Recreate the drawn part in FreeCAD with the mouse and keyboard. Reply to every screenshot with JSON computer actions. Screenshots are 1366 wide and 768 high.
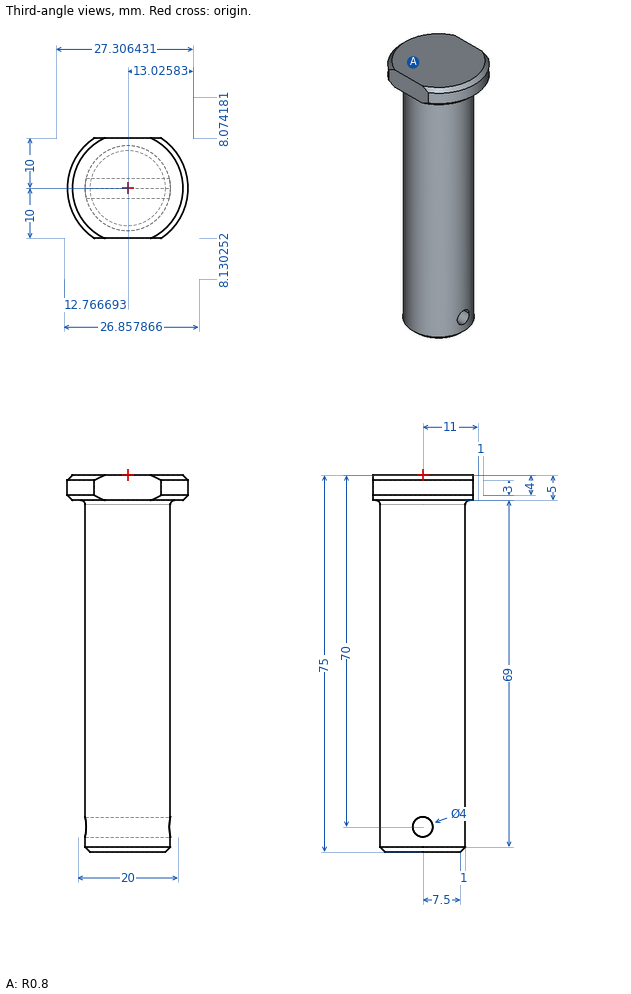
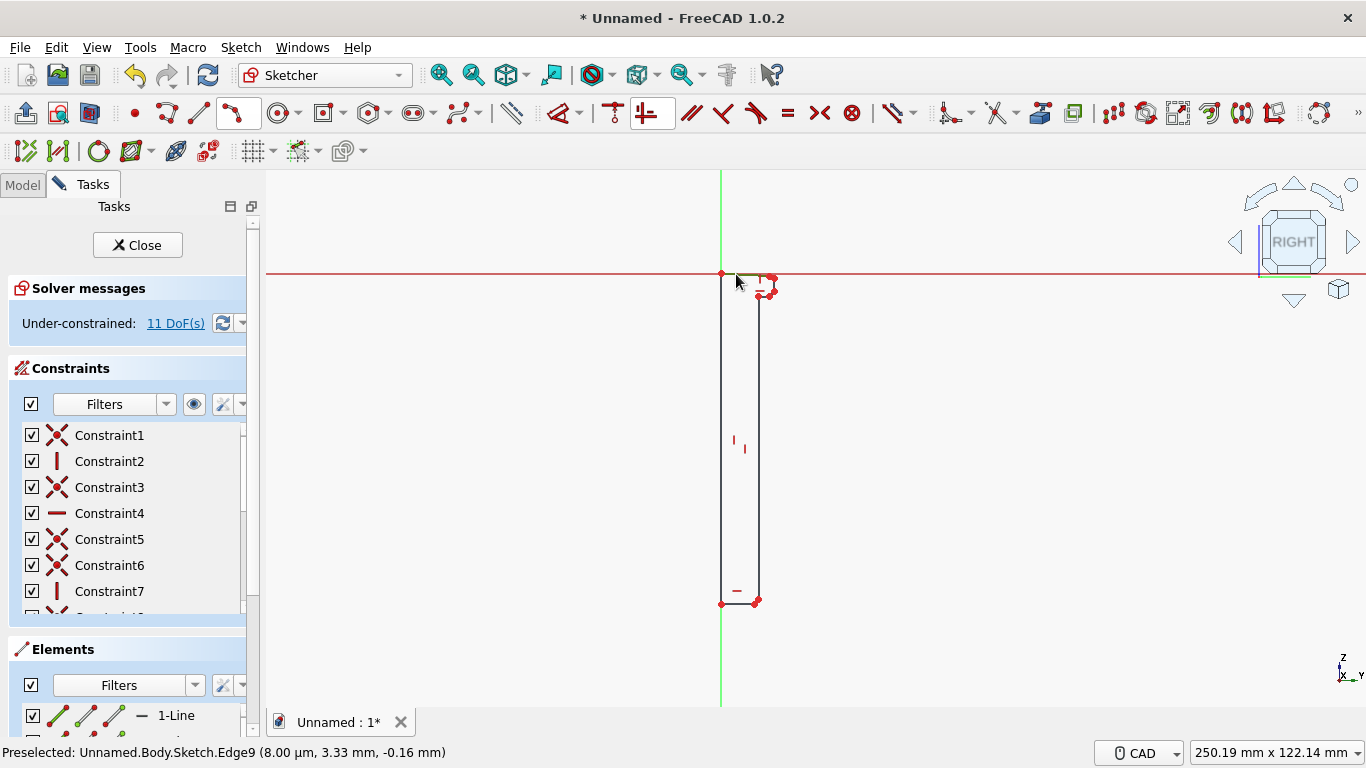
{"action": "key", "text": "h"}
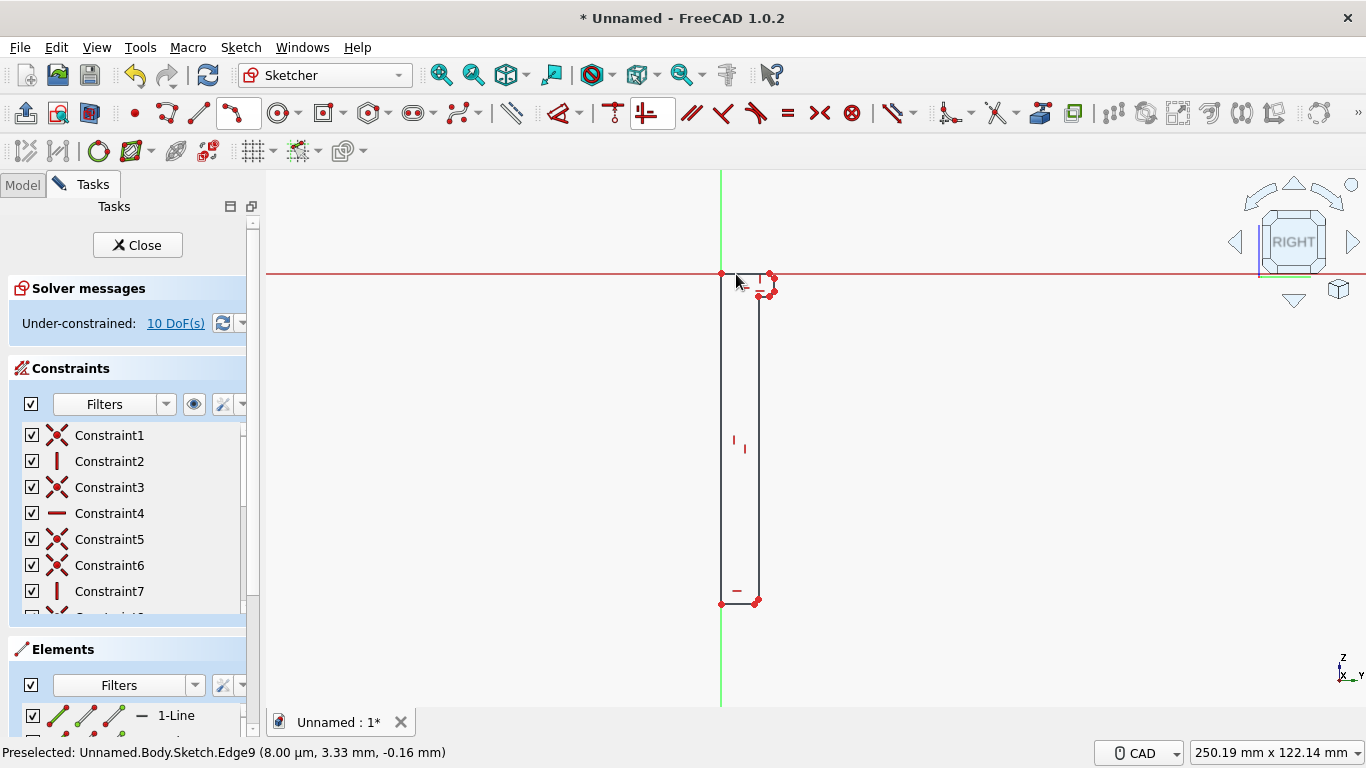
{"action": "left_click", "coordinate": [558, 114]}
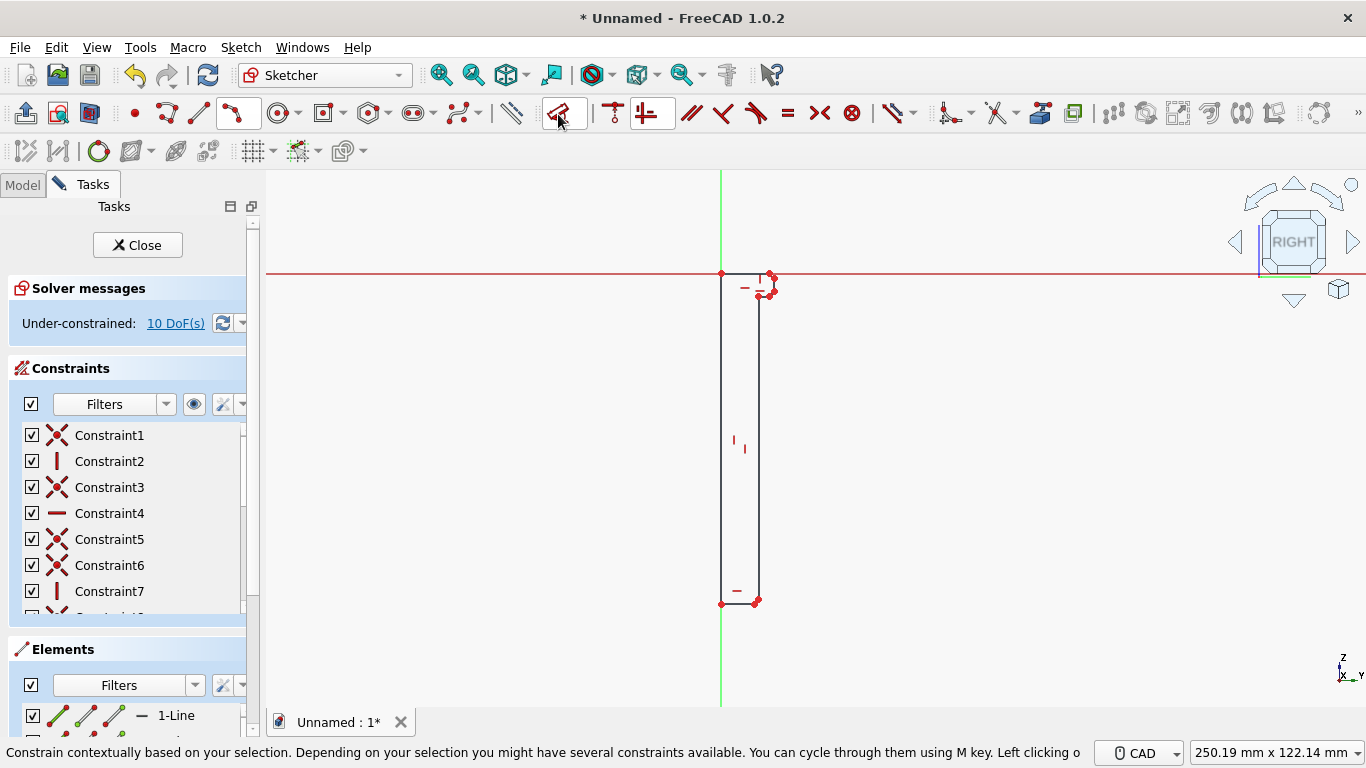
{"action": "scroll", "coordinate": [774, 285], "scroll_direction": "up", "scroll_amount": 6}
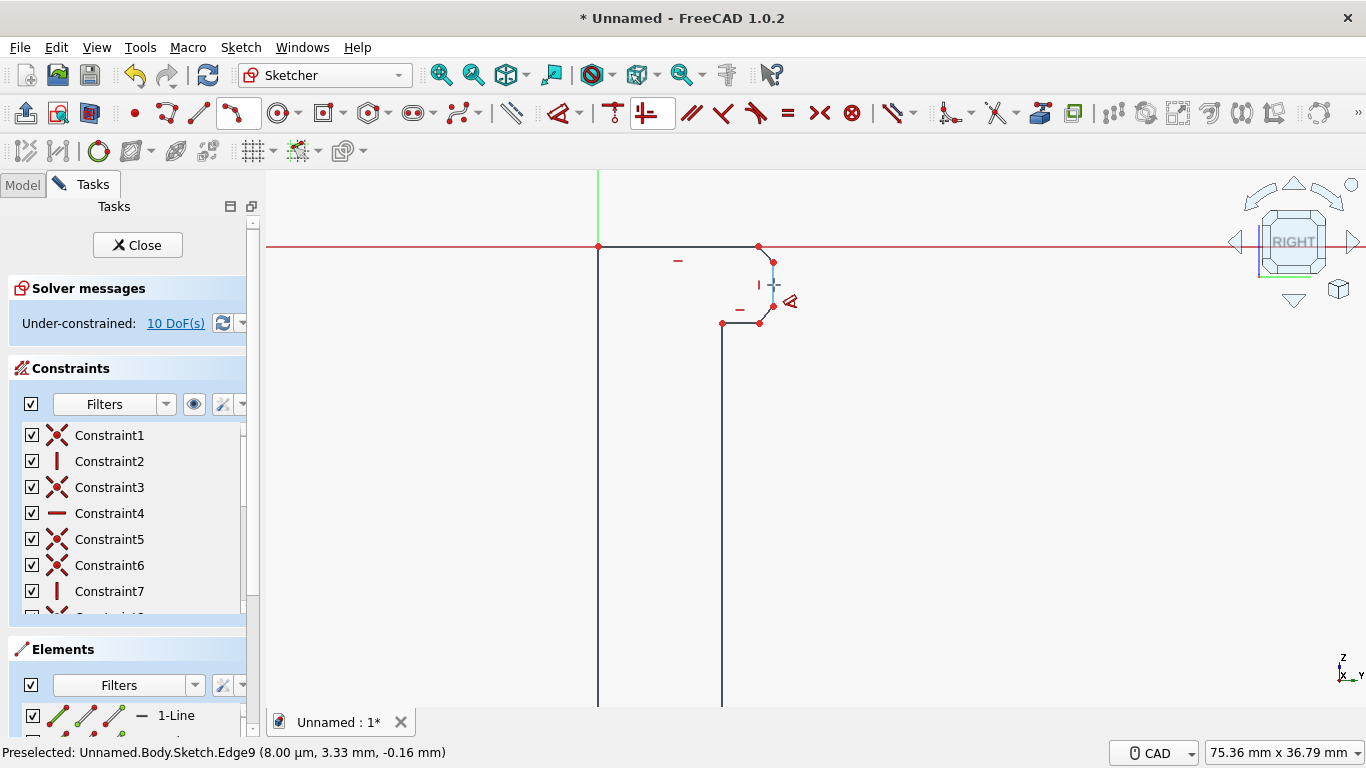
{"action": "left_click", "coordinate": [773, 284]}
{"action": "left_click", "coordinate": [807, 284]}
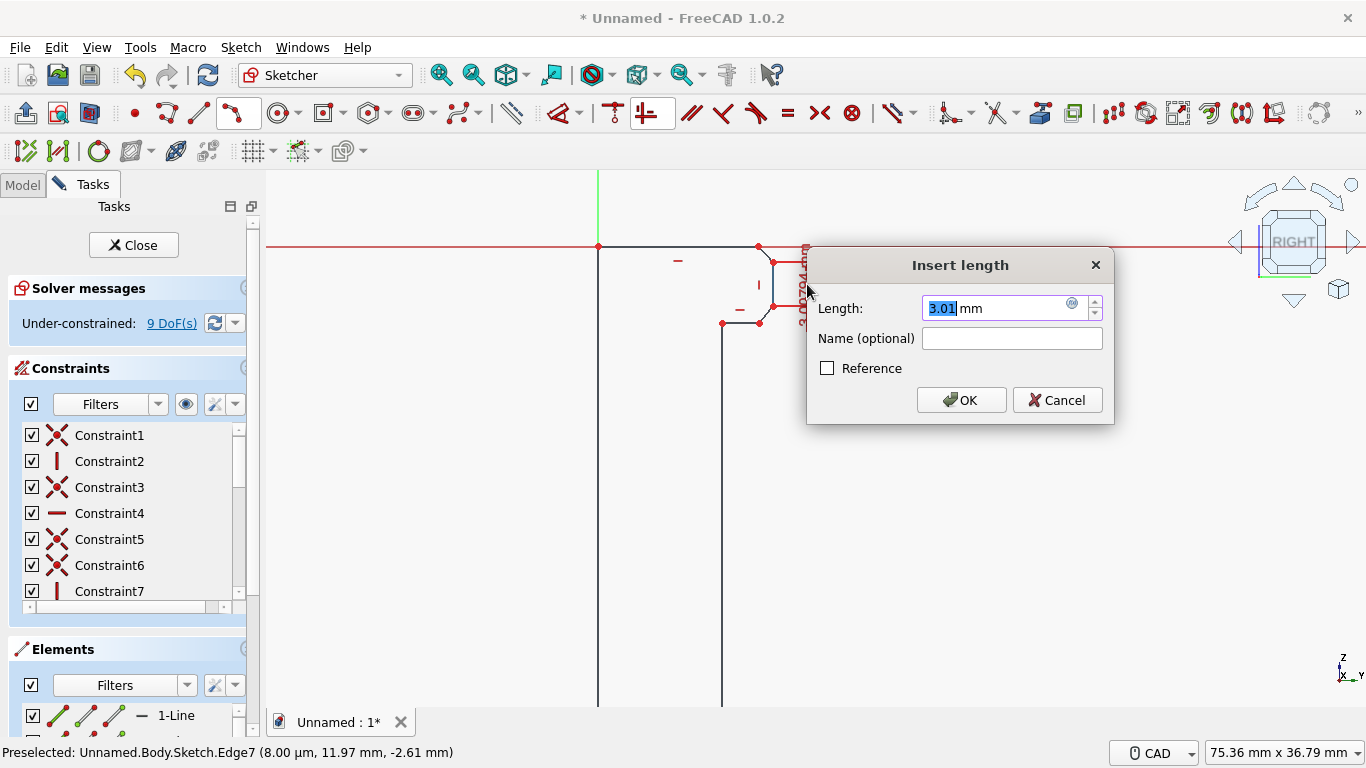
{"action": "type", "text": "3"}
{"action": "key", "text": "Return"}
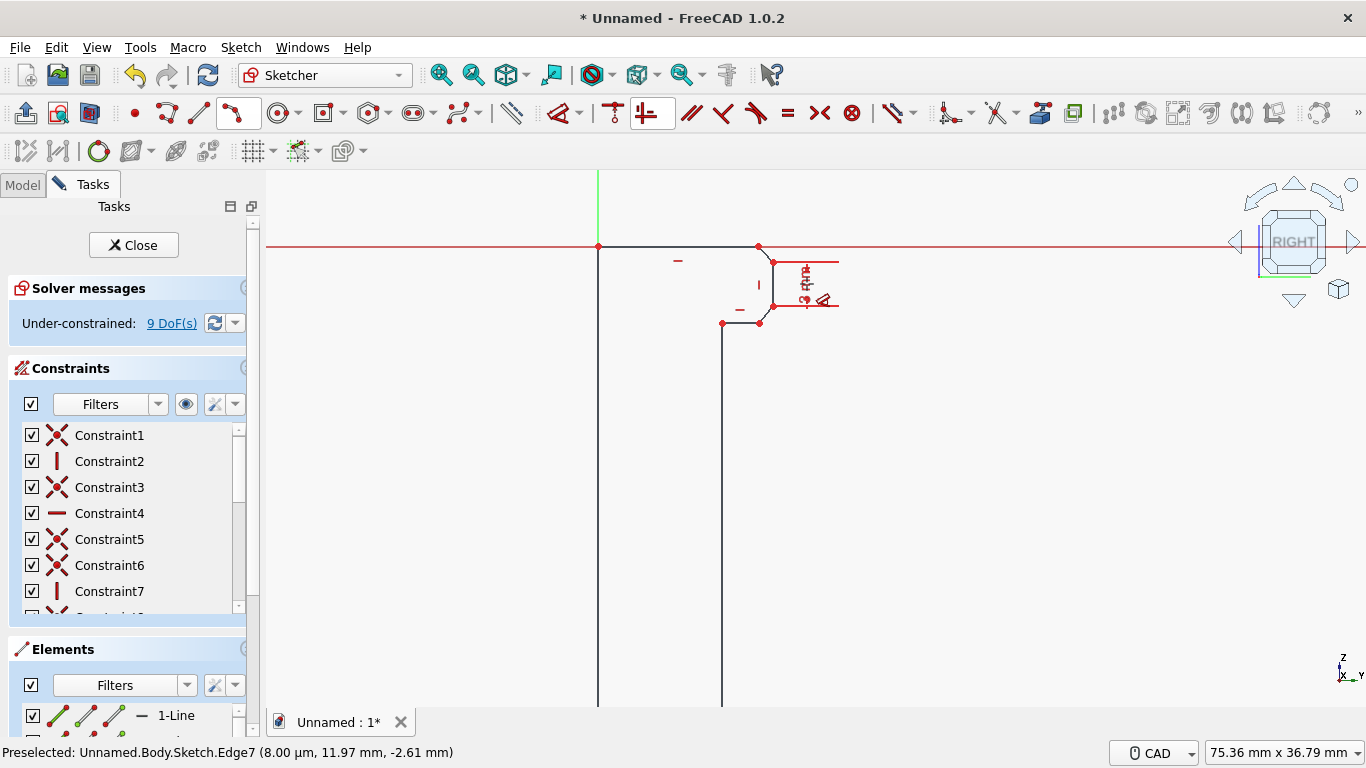
{"action": "scroll", "coordinate": [774, 285], "scroll_direction": "down", "scroll_amount": 6}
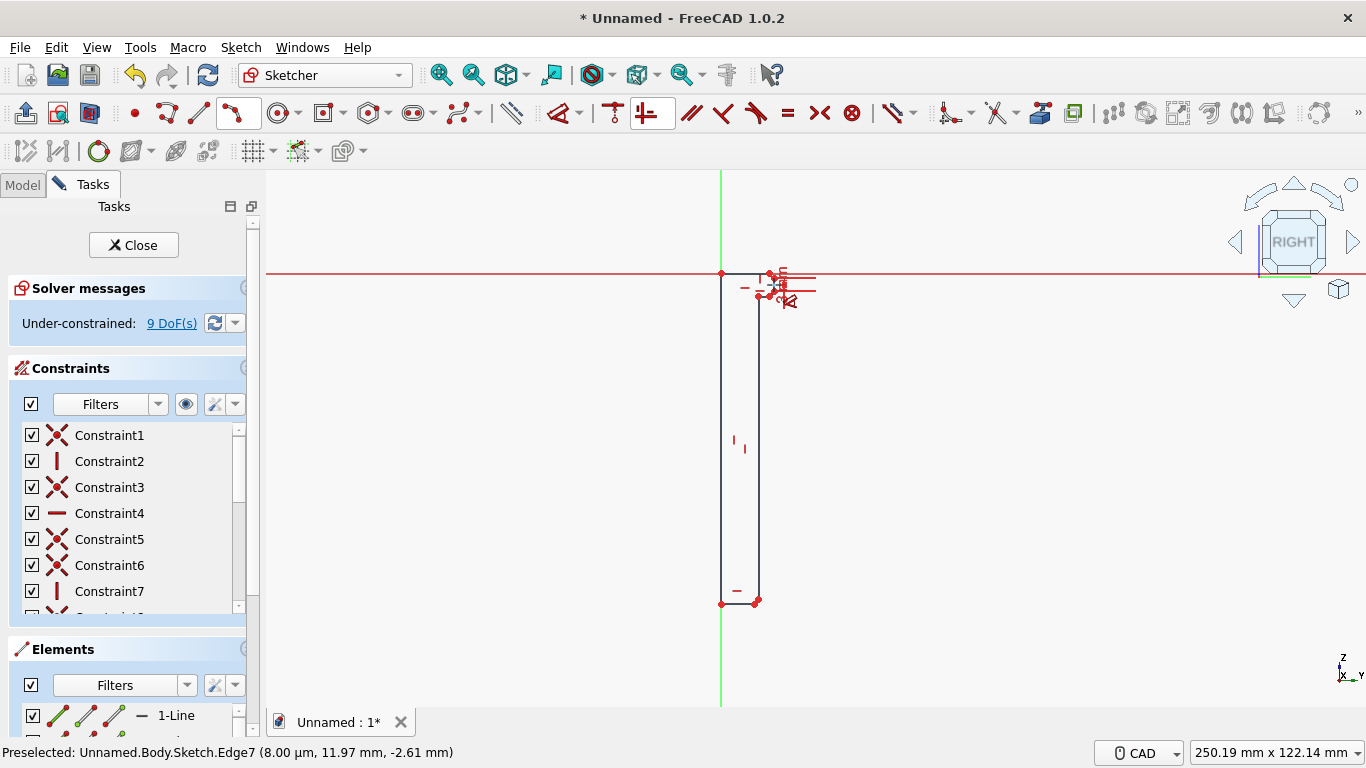
{"action": "left_click", "coordinate": [721, 373]}
{"action": "left_click", "coordinate": [687, 439]}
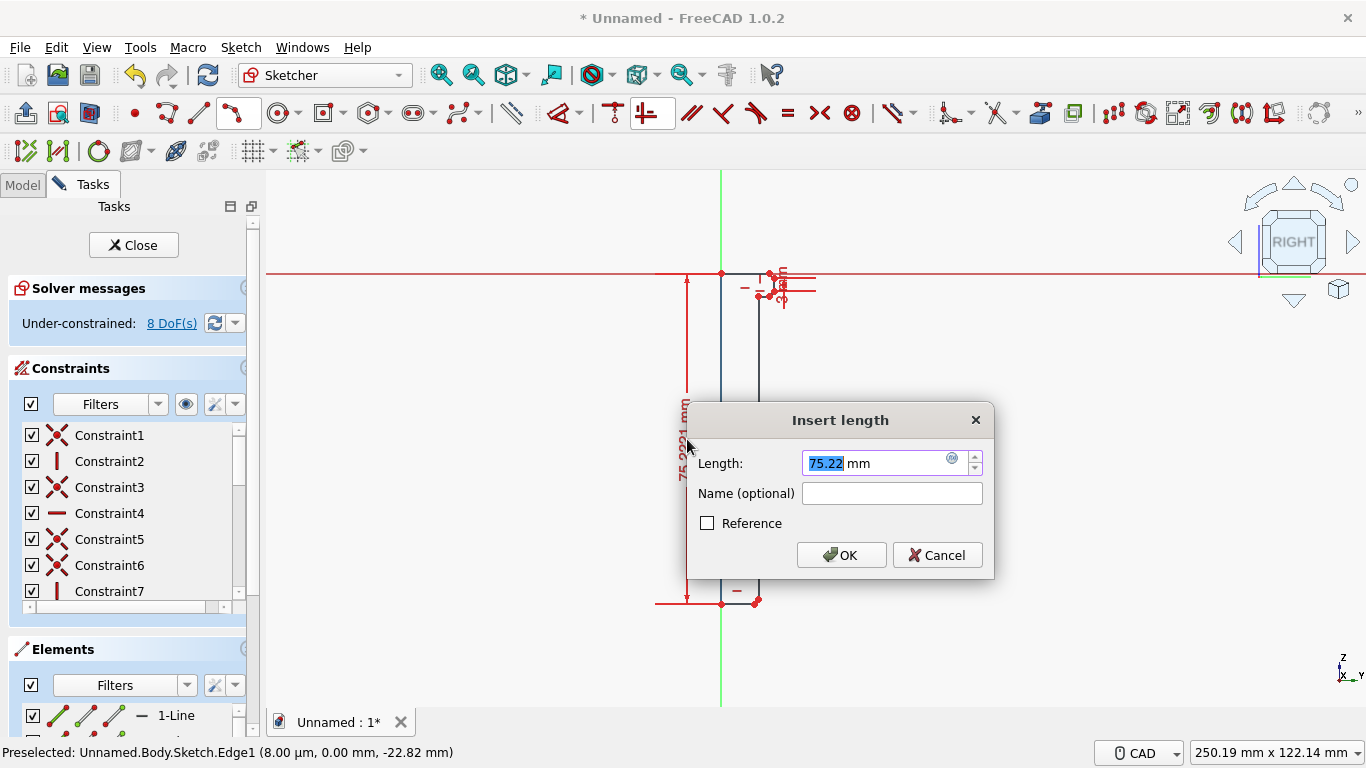
{"action": "type", "text": "75"}
{"action": "key", "text": "Return"}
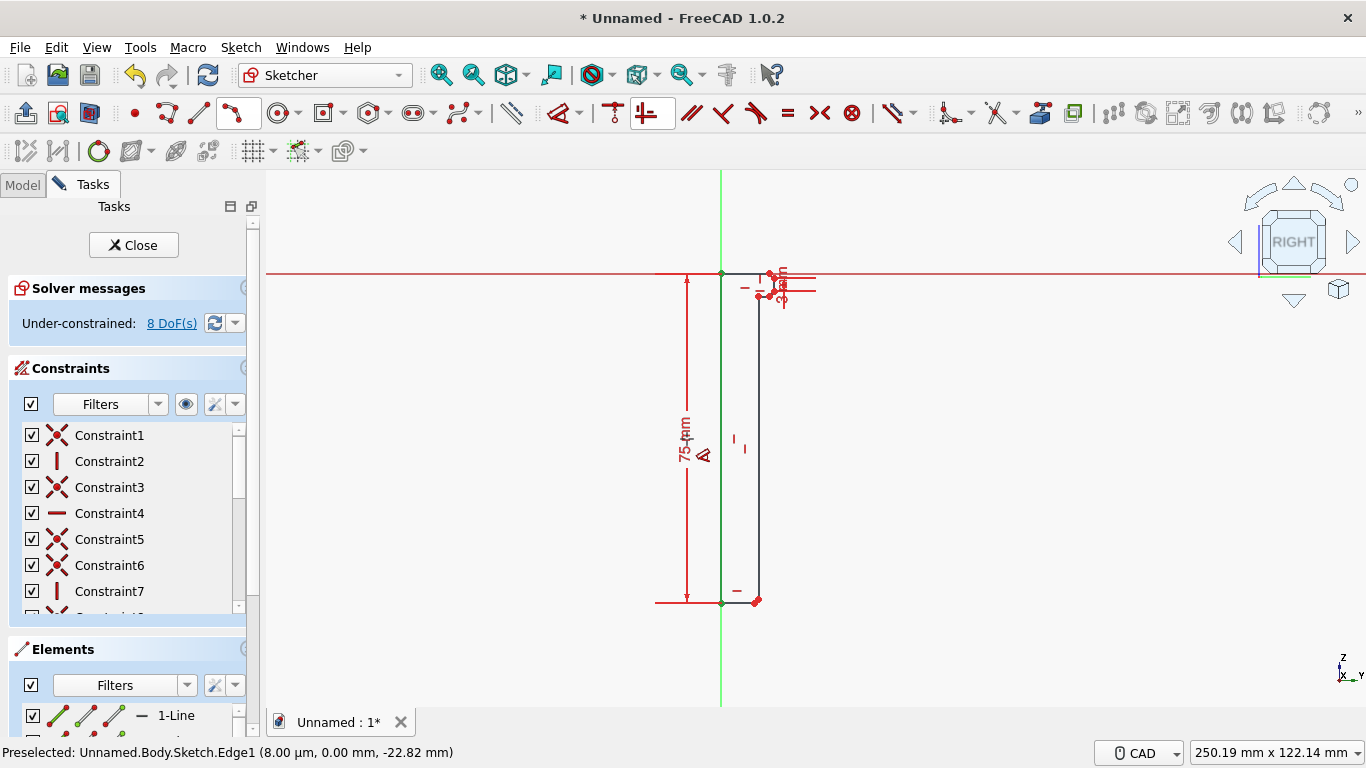
{"action": "left_click", "coordinate": [759, 509]}
{"action": "left_click", "coordinate": [793, 448]}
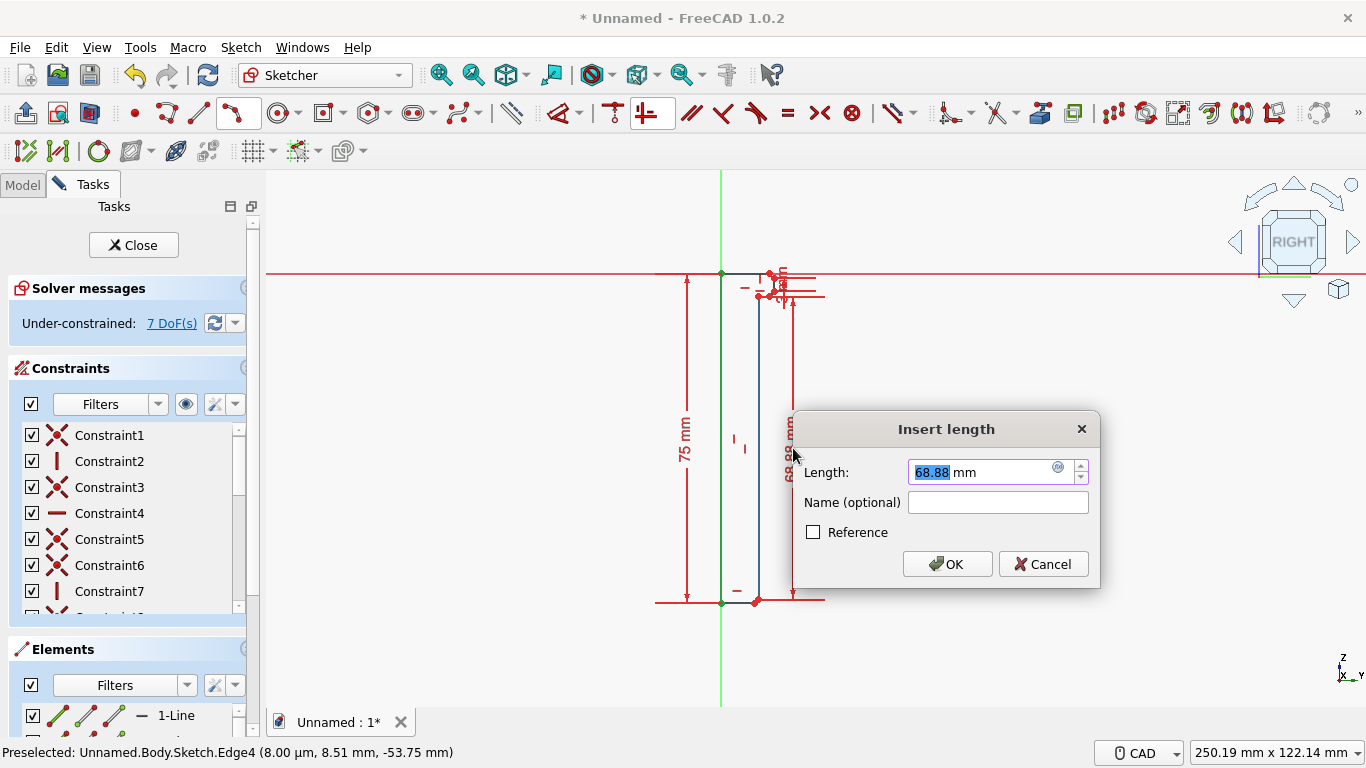
{"action": "type", "text": "69"}
{"action": "key", "text": "Return"}